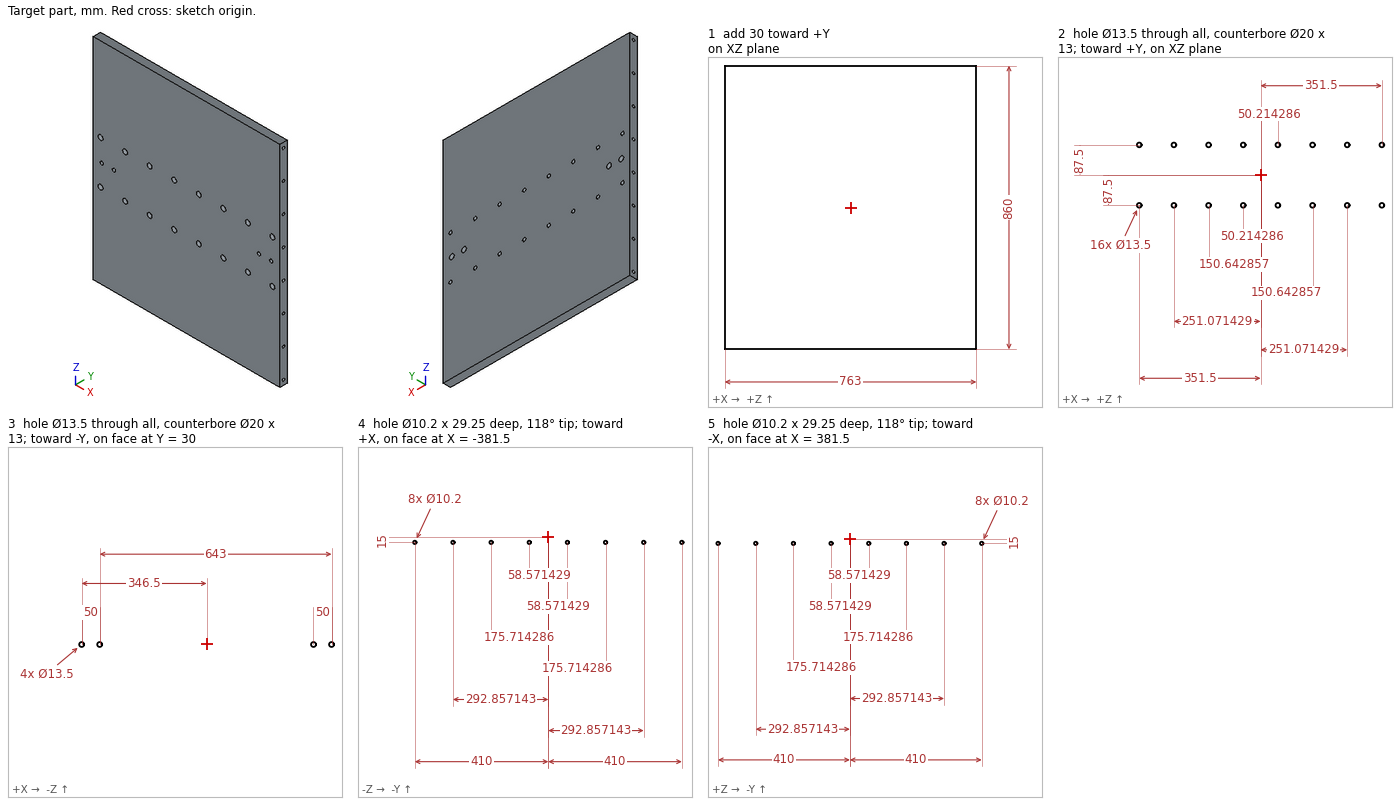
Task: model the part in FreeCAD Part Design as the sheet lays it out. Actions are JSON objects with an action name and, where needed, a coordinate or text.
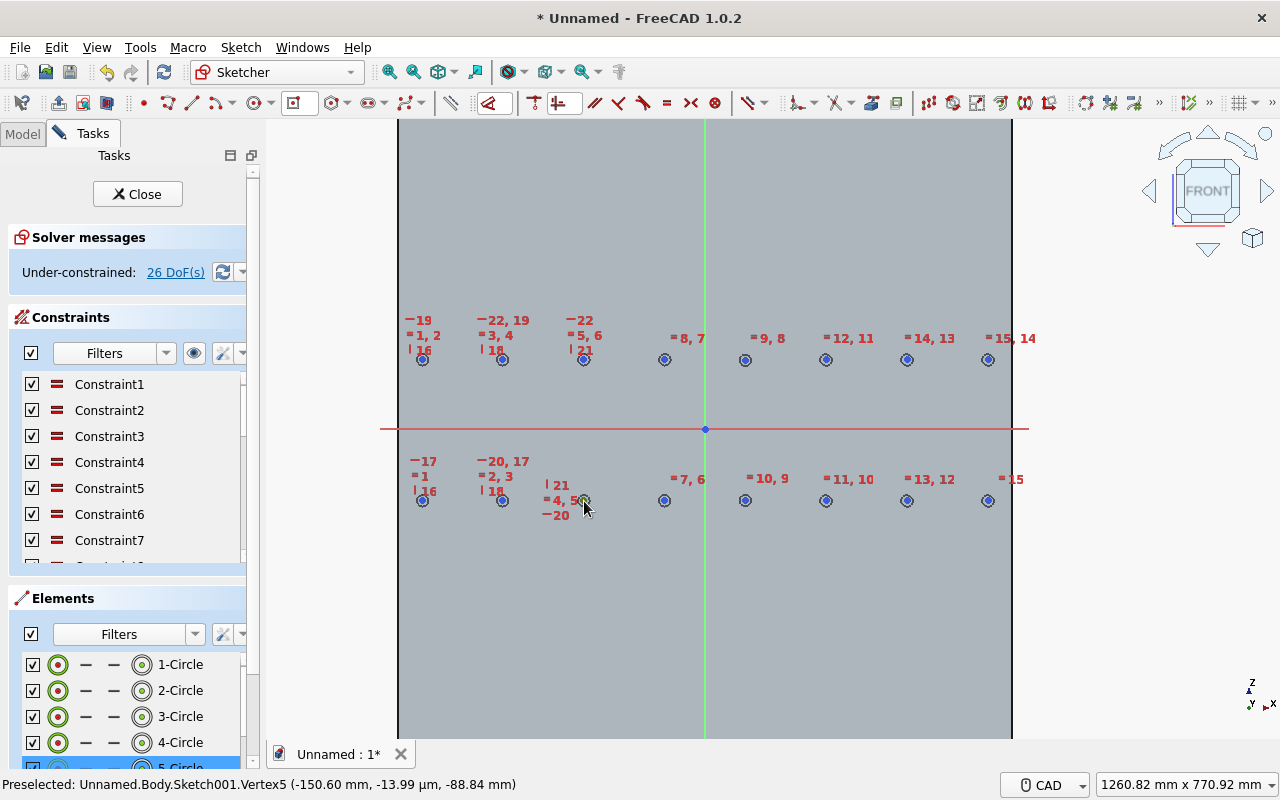
{"action": "left_click", "coordinate": [665, 501]}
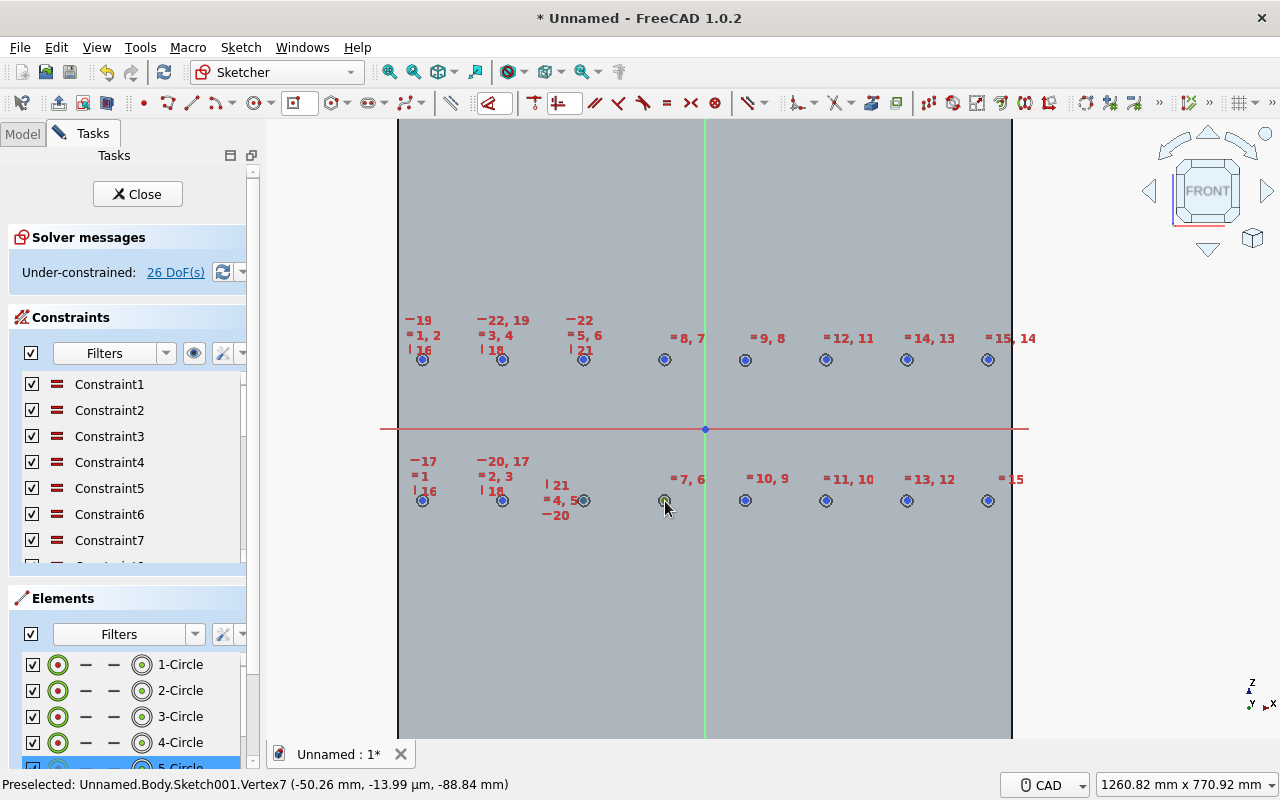
{"action": "left_click", "coordinate": [576, 104]}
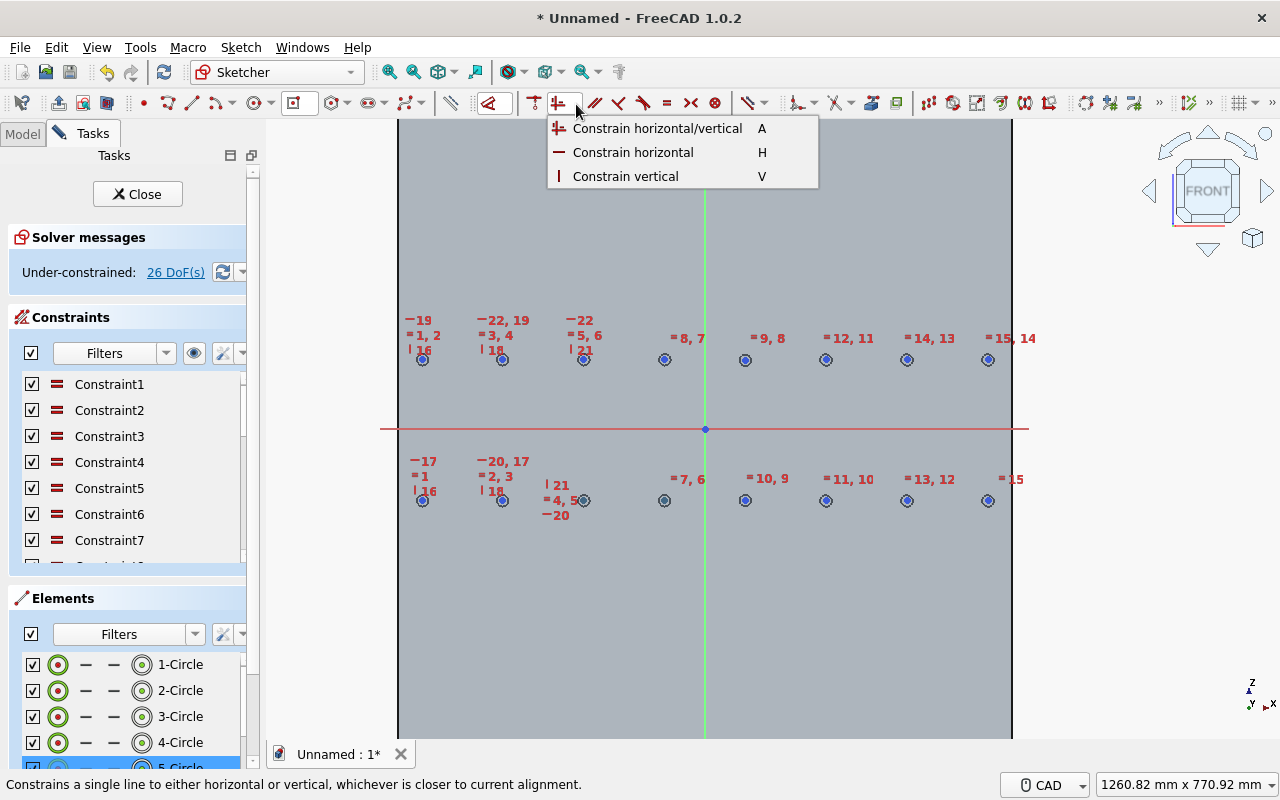
{"action": "left_click", "coordinate": [683, 152]}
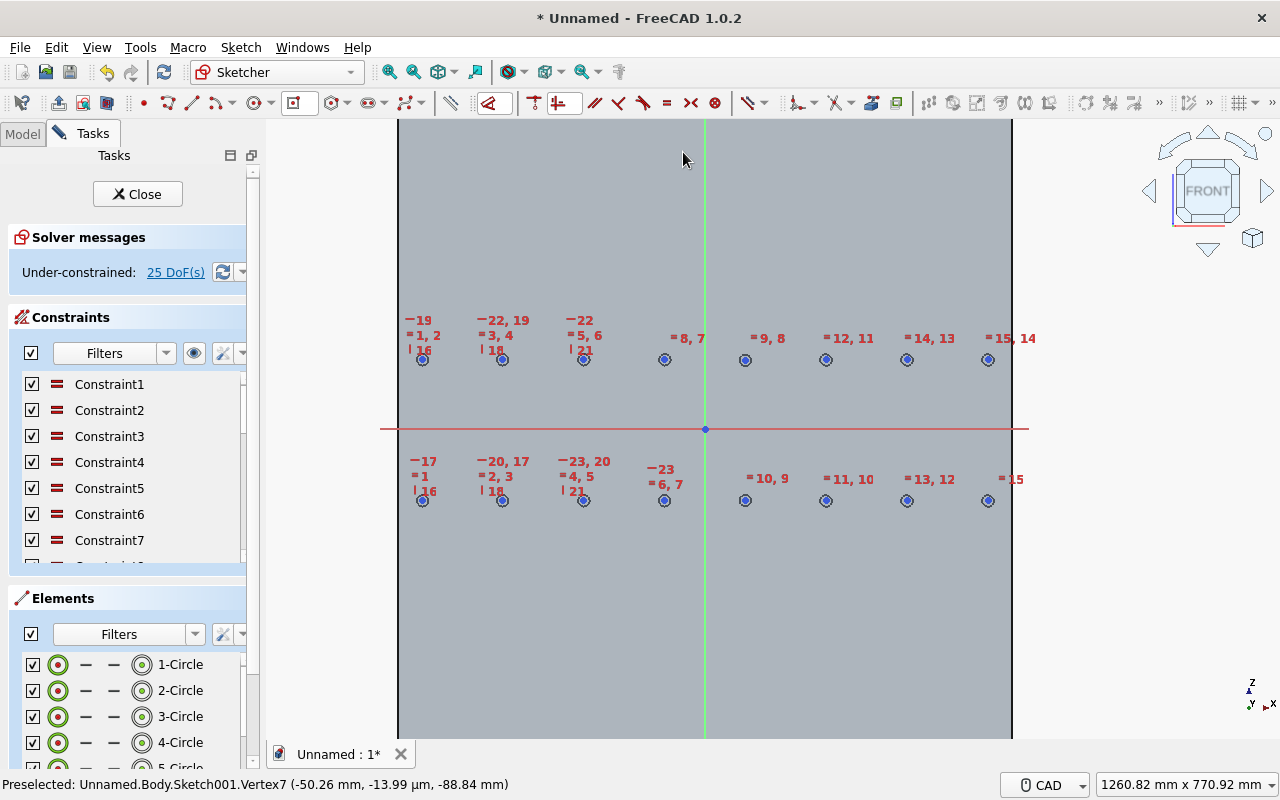
{"action": "left_click", "coordinate": [665, 501]}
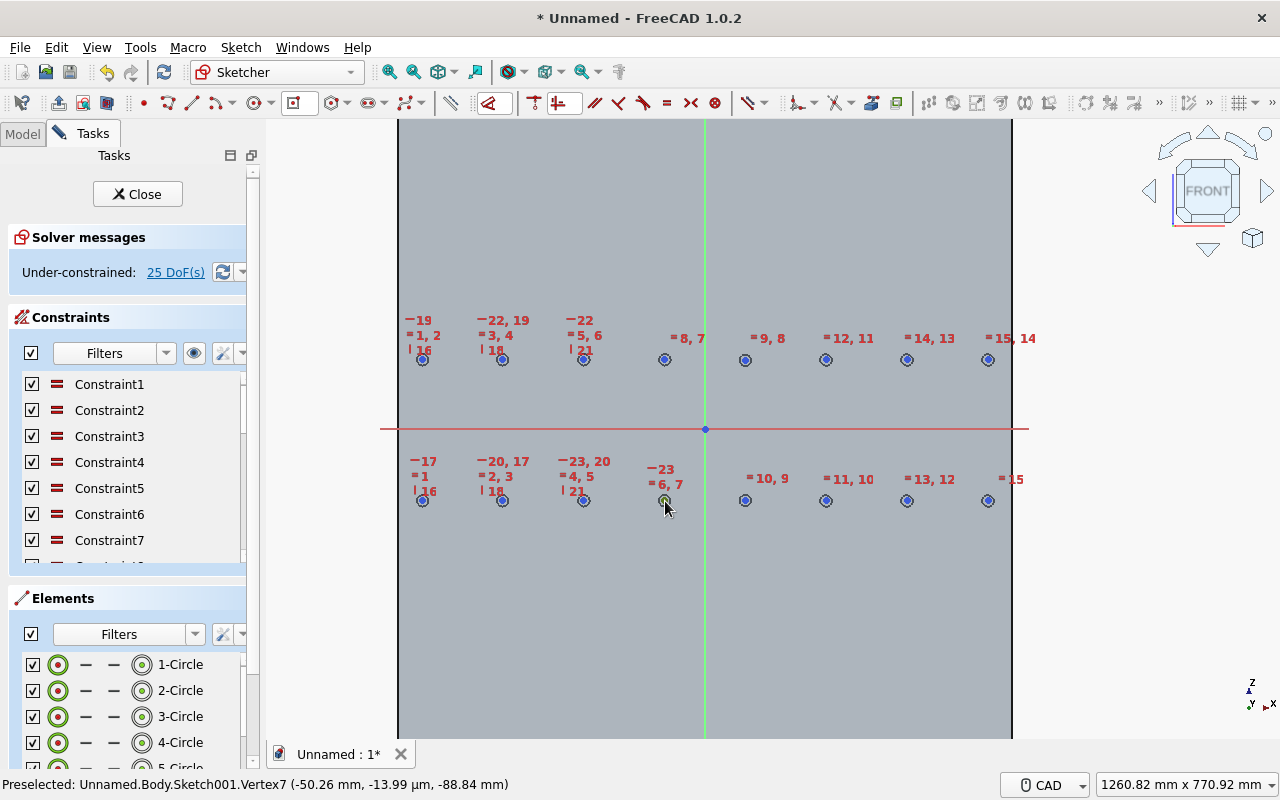
{"action": "left_click", "coordinate": [665, 360]}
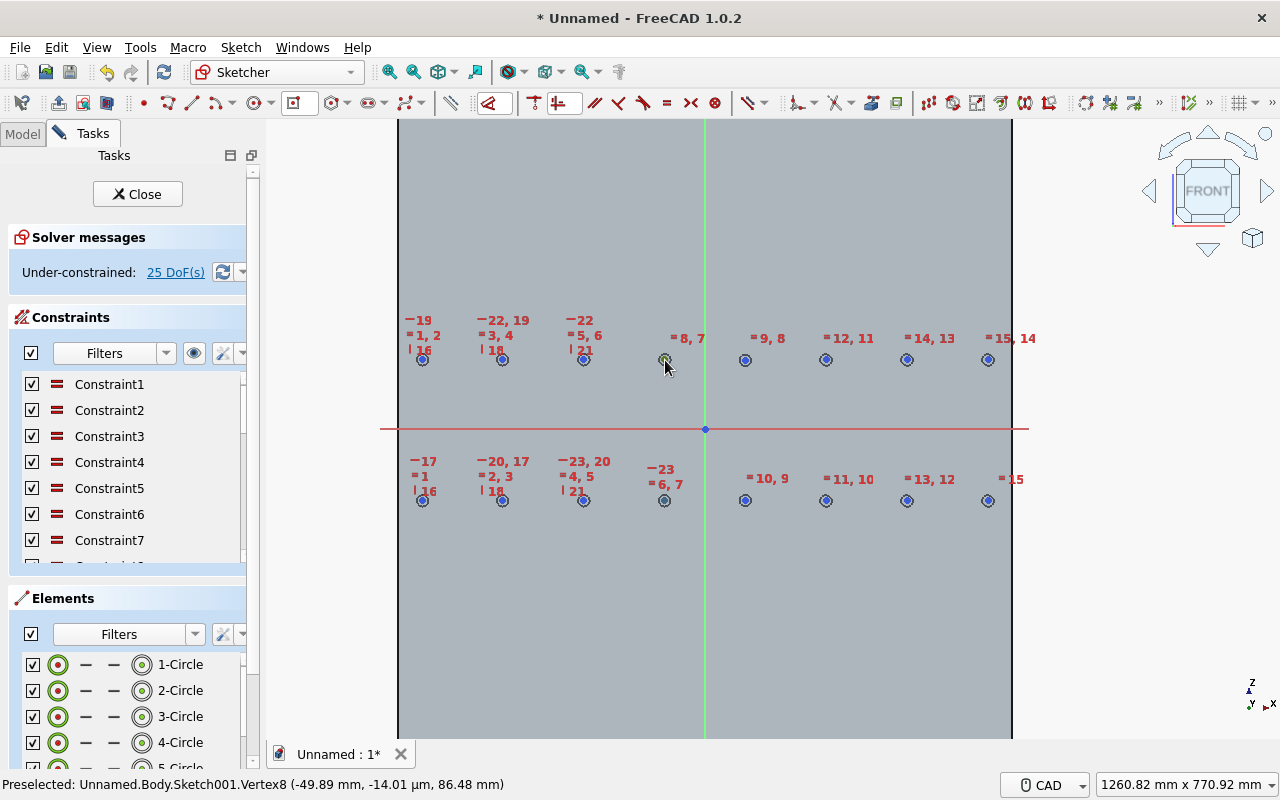
{"action": "left_click", "coordinate": [576, 104]}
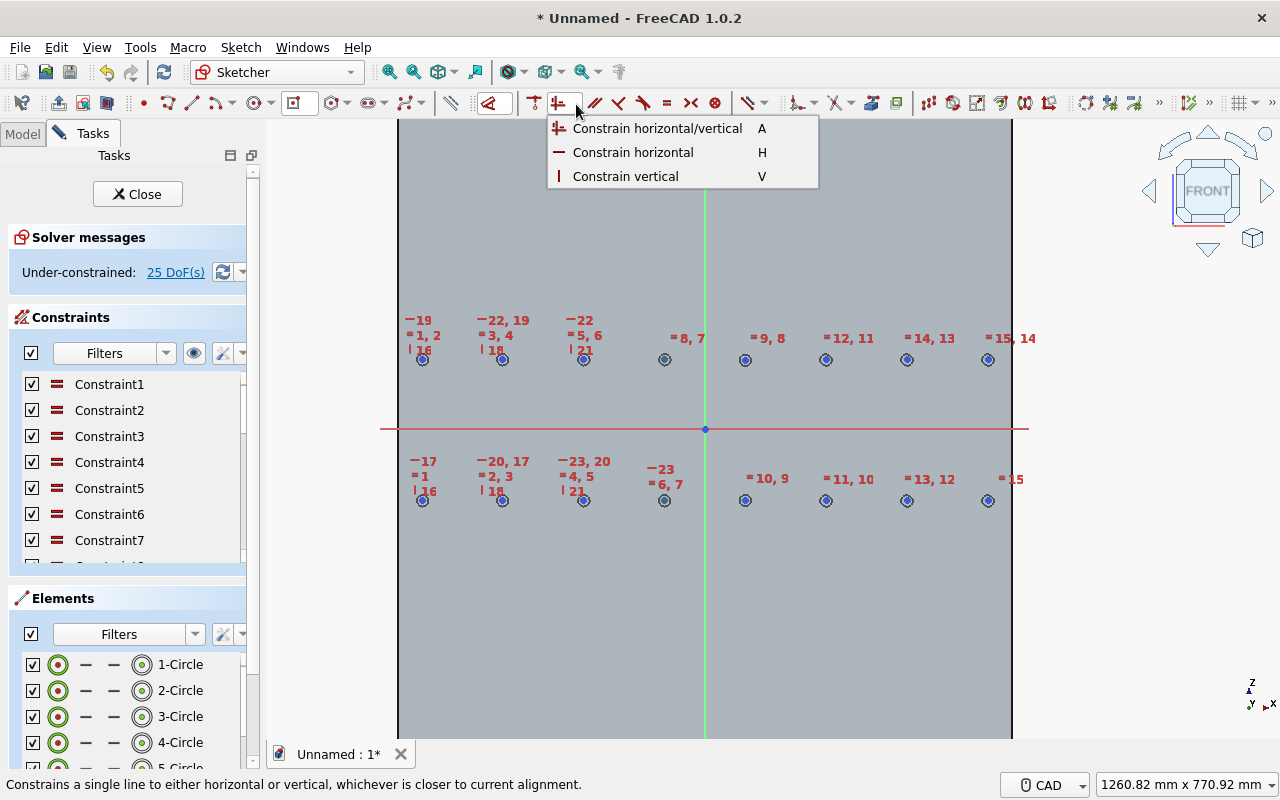
{"action": "left_click", "coordinate": [683, 176]}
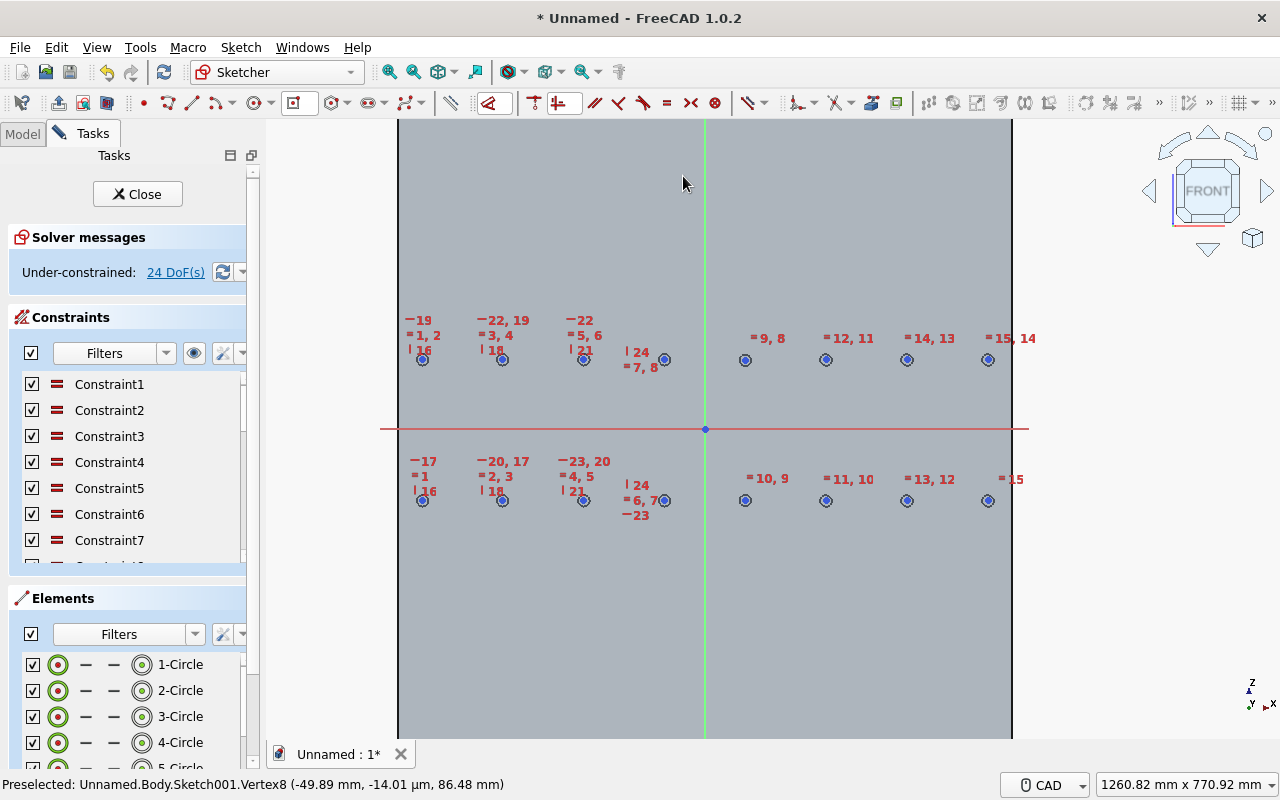
{"action": "left_click", "coordinate": [584, 360]}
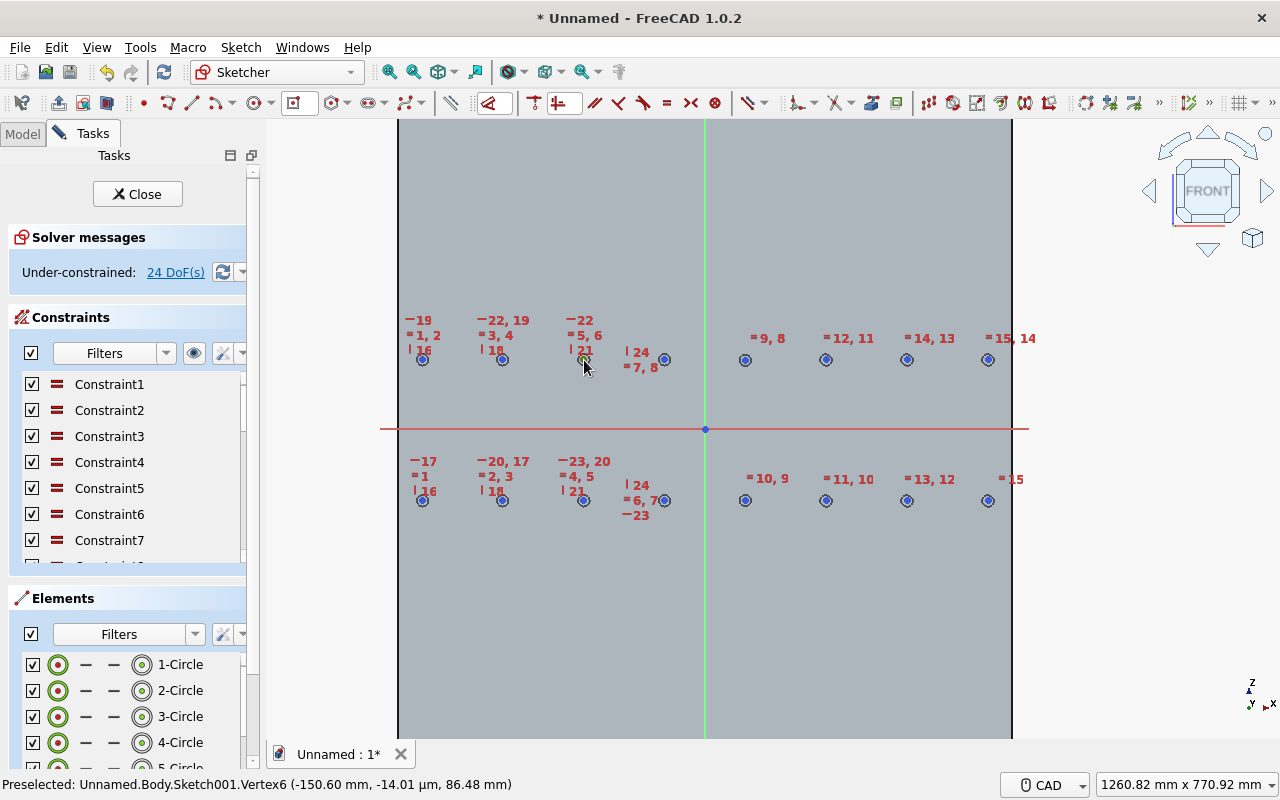
{"action": "left_click", "coordinate": [665, 360]}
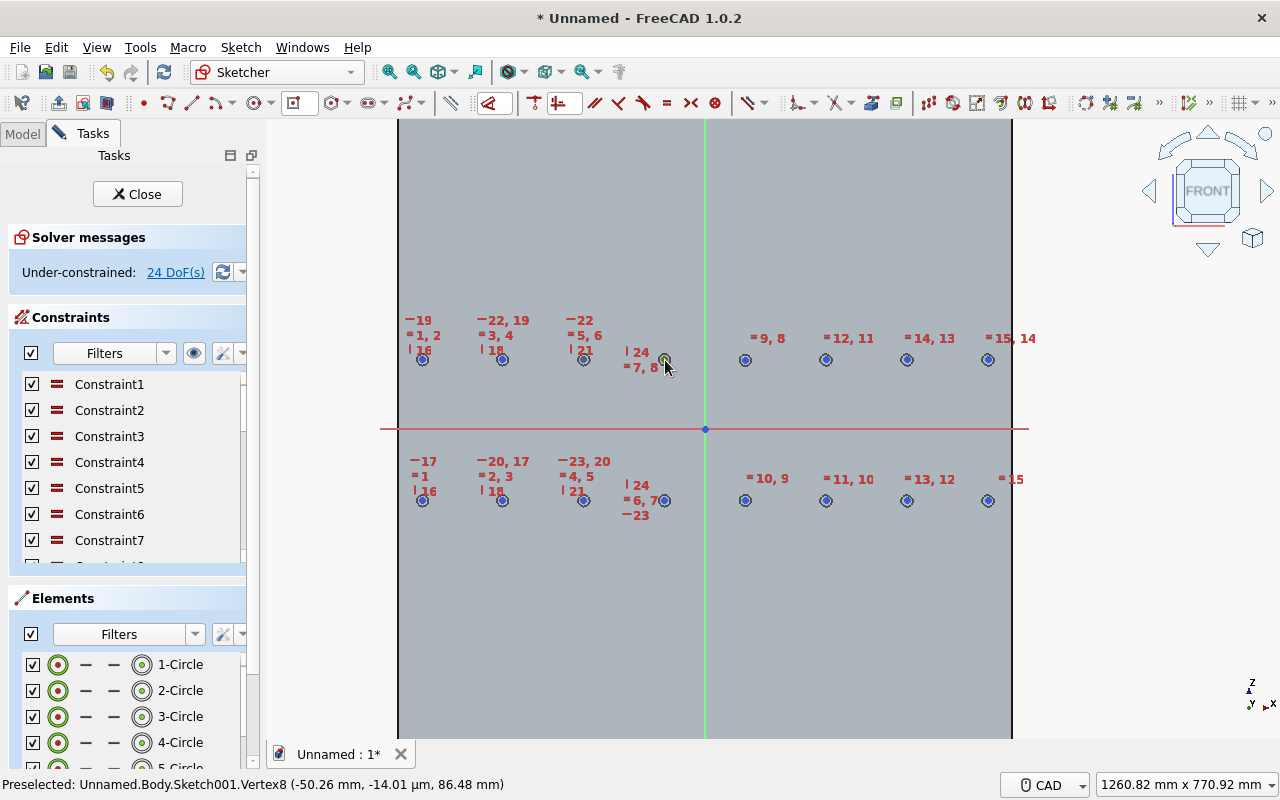
{"action": "left_click", "coordinate": [576, 104]}